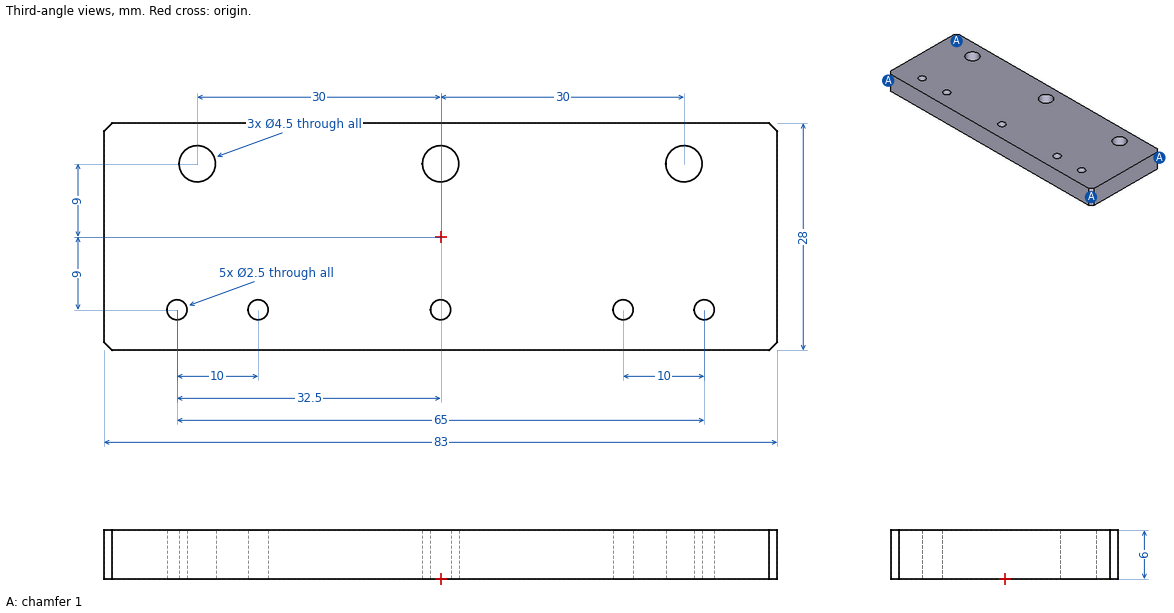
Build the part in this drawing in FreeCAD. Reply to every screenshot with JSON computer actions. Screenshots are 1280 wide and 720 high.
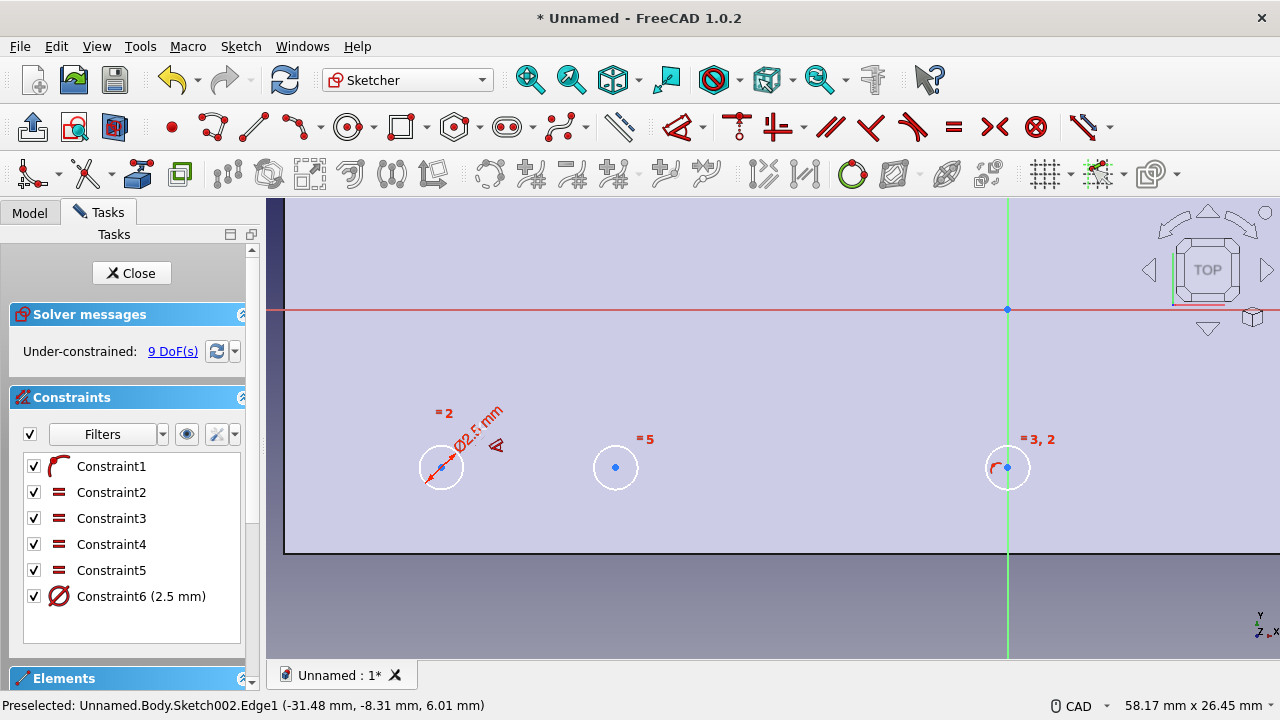
{"action": "left_click", "coordinate": [441, 468]}
{"action": "left_click", "coordinate": [407, 389]}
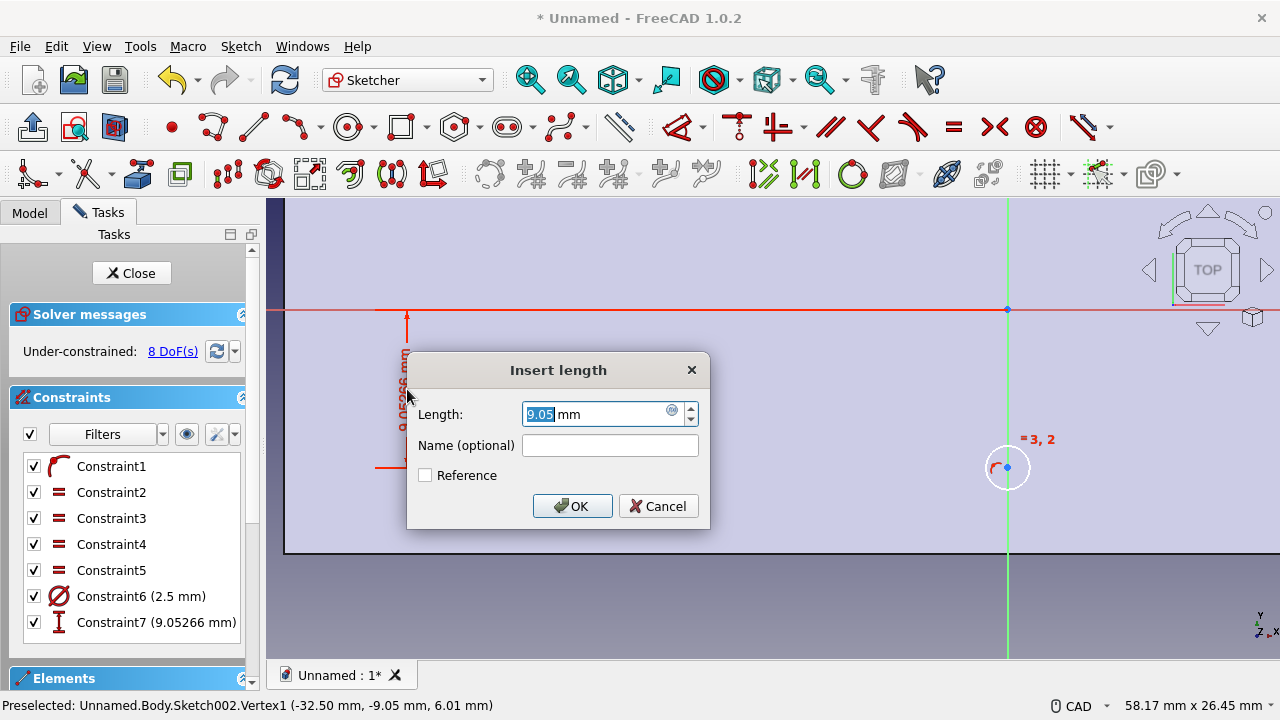
{"action": "type", "text": "9"}
{"action": "key", "text": "Return"}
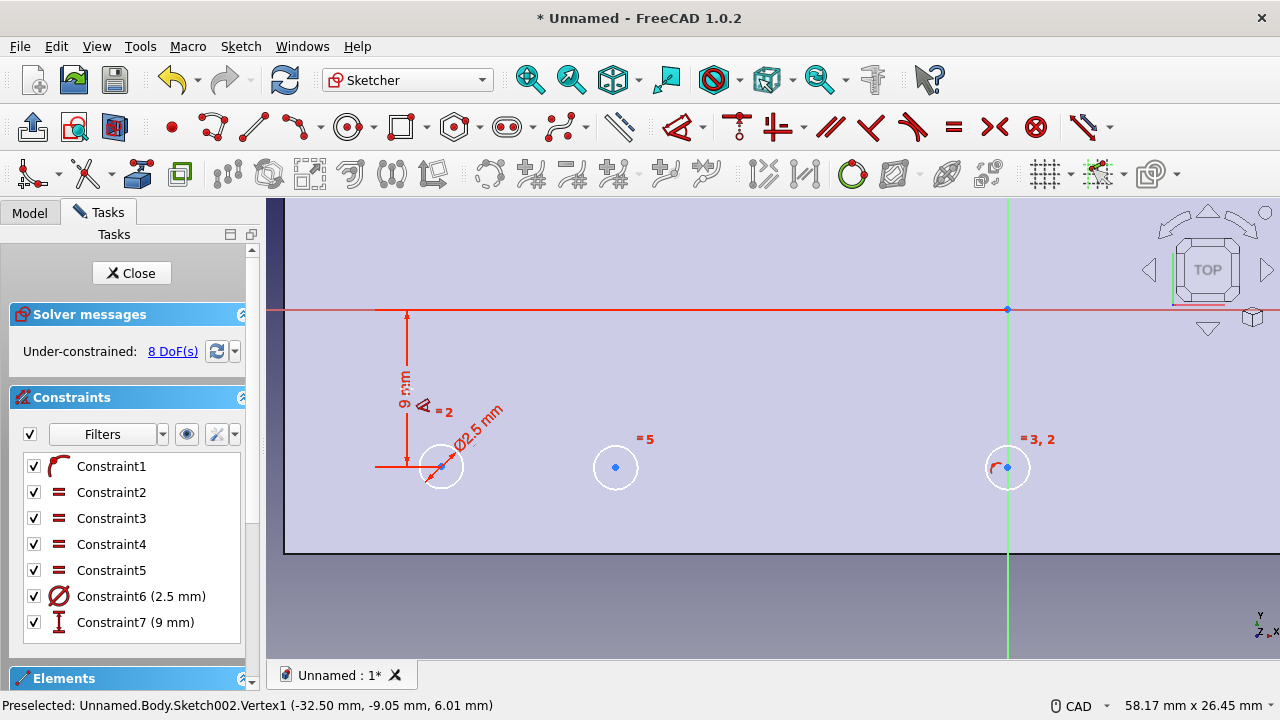
{"action": "left_click", "coordinate": [1008, 468]}
{"action": "left_click", "coordinate": [1042, 389]}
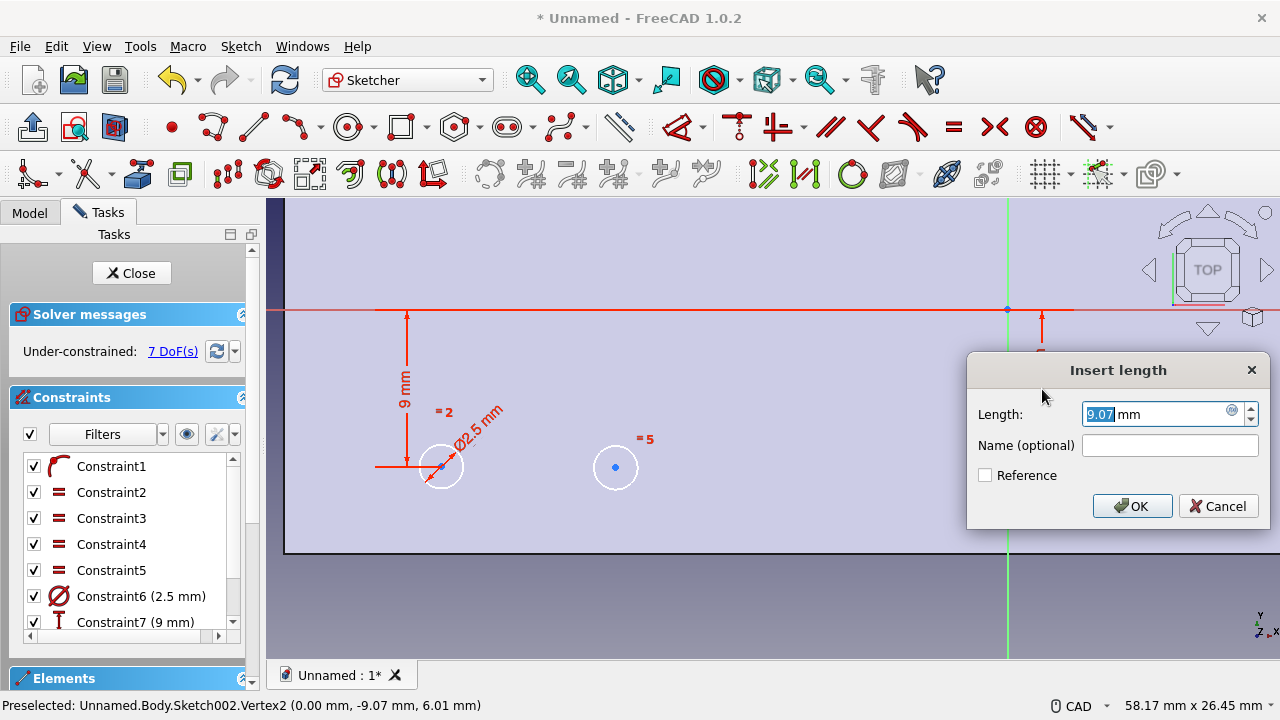
{"action": "type", "text": "9"}
{"action": "key", "text": "Return"}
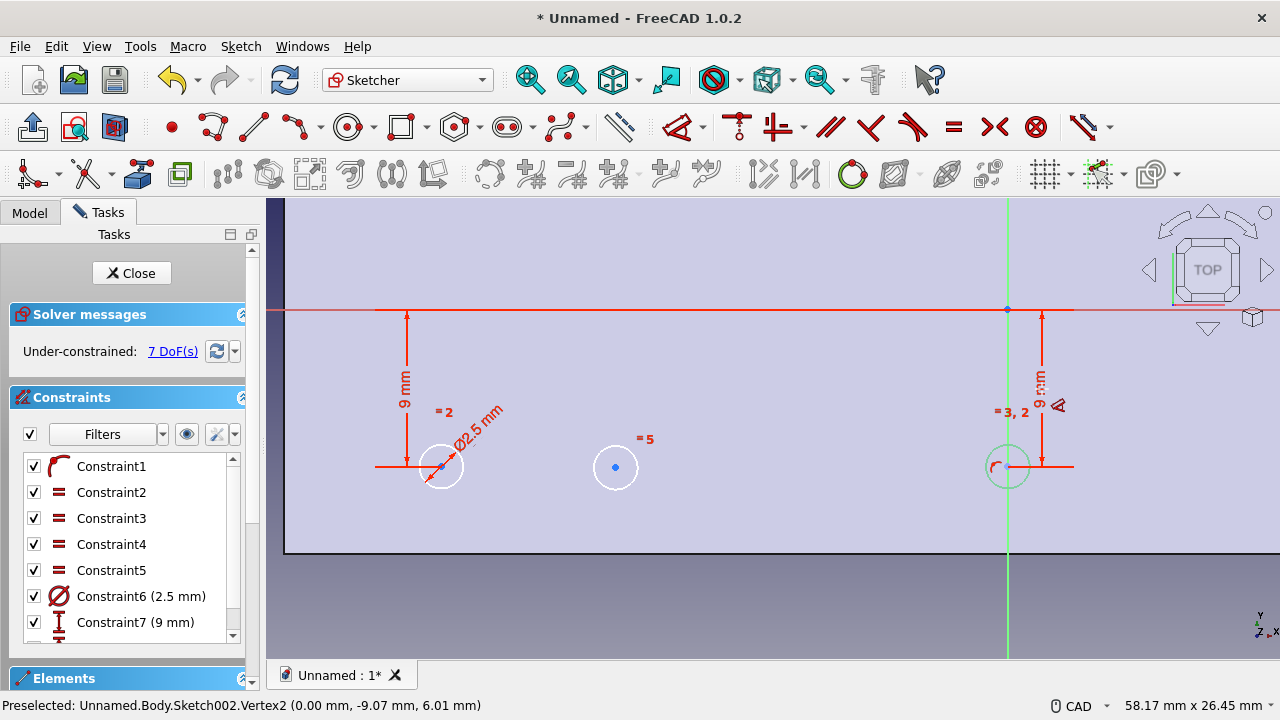
{"action": "scroll", "coordinate": [457, 452], "scroll_direction": "down", "scroll_amount": 4}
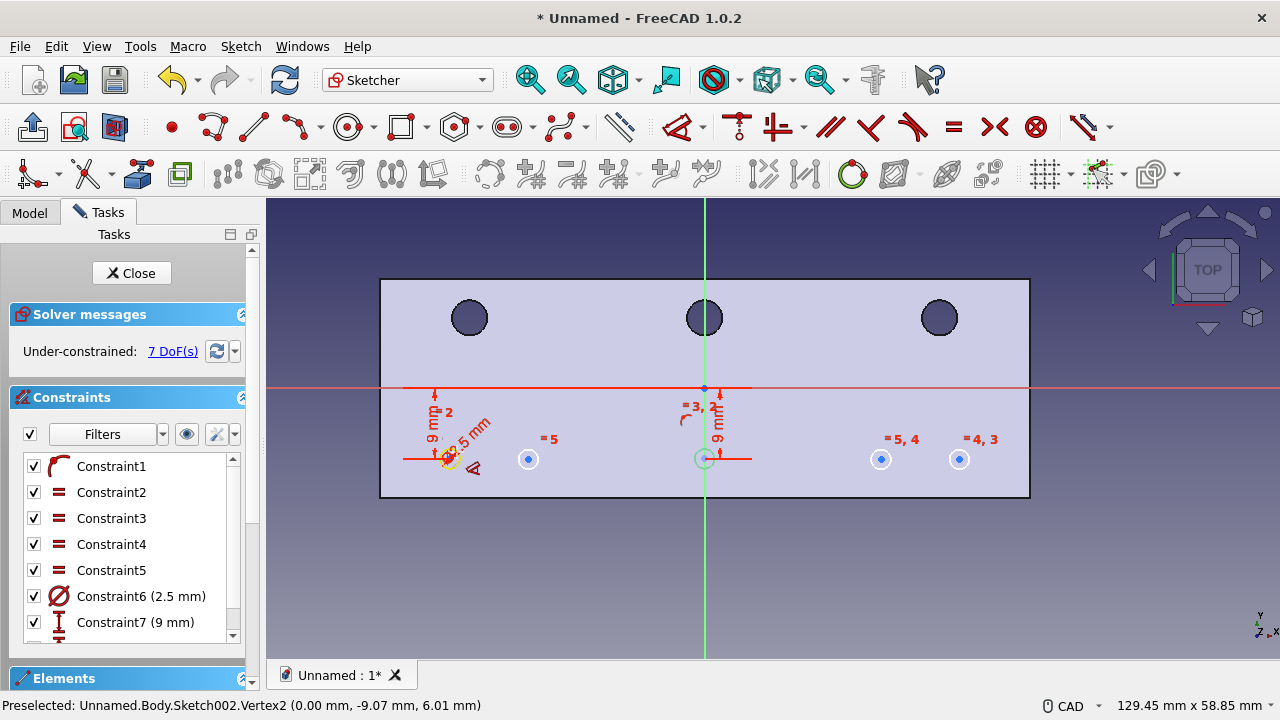
{"action": "left_click", "coordinate": [959, 459]}
{"action": "left_click", "coordinate": [993, 424]}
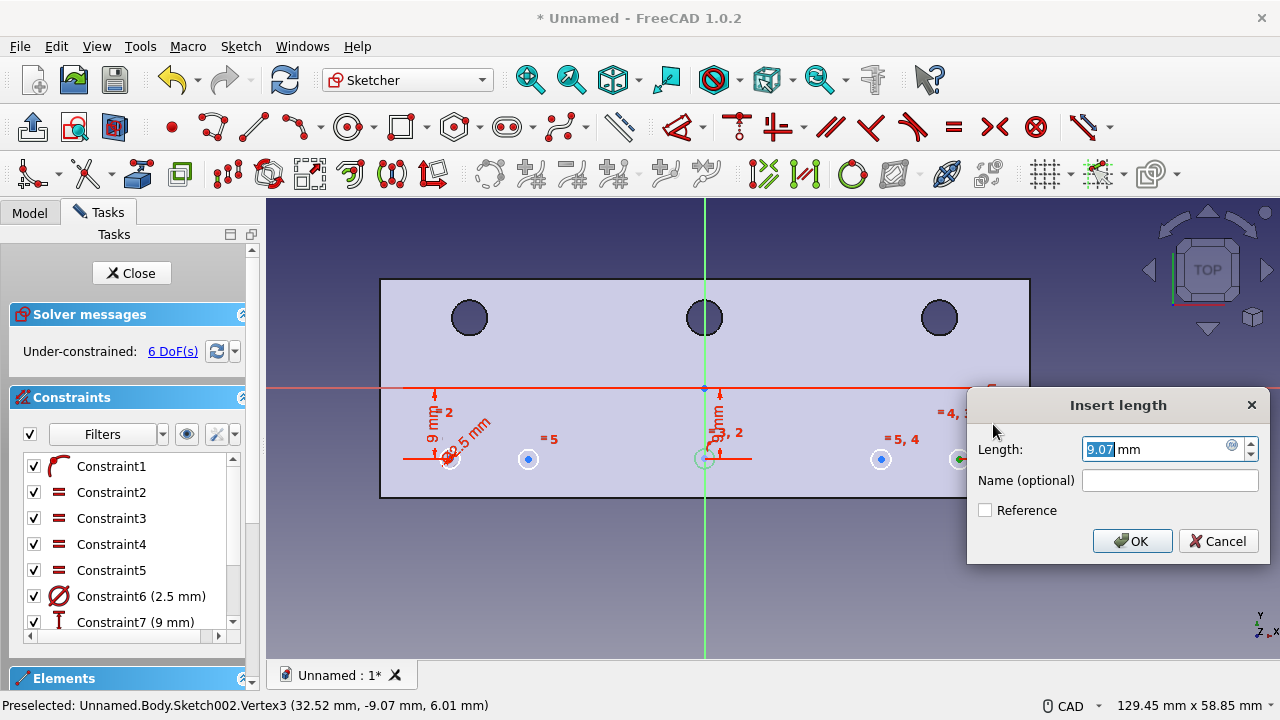
{"action": "type", "text": "9"}
{"action": "key", "text": "Return"}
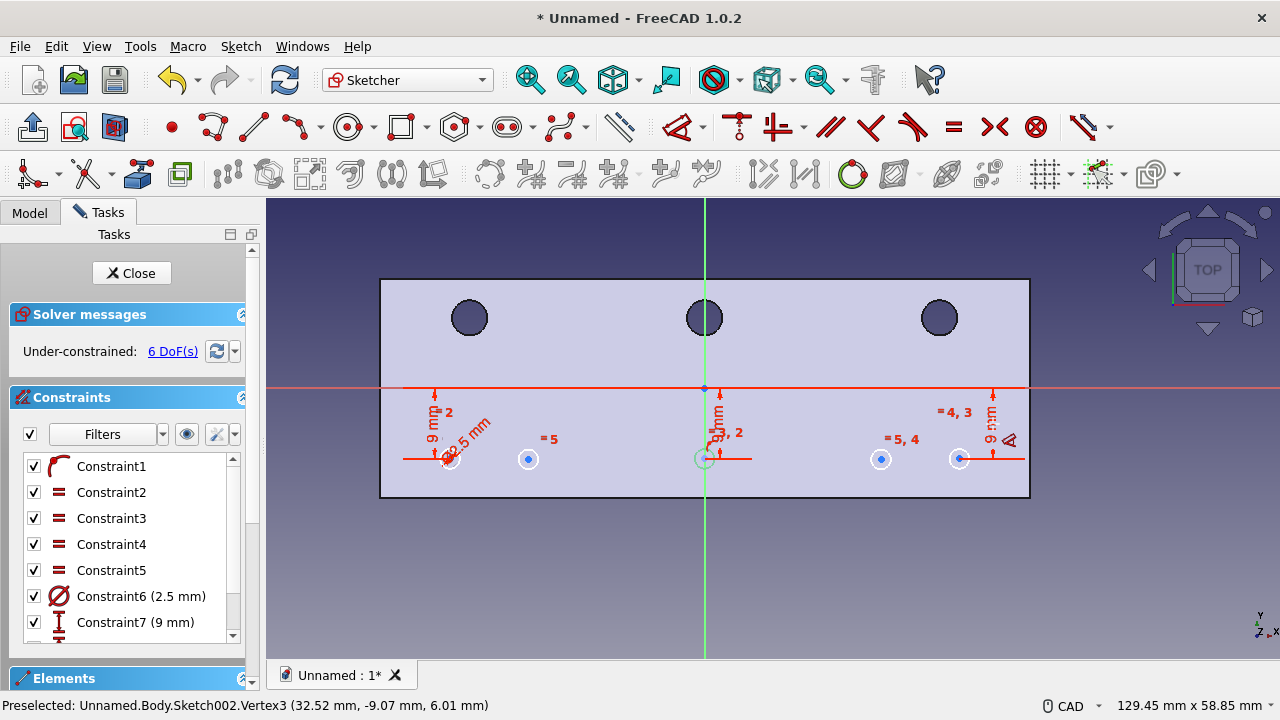
{"action": "left_click", "coordinate": [881, 459]}
{"action": "left_click", "coordinate": [915, 424]}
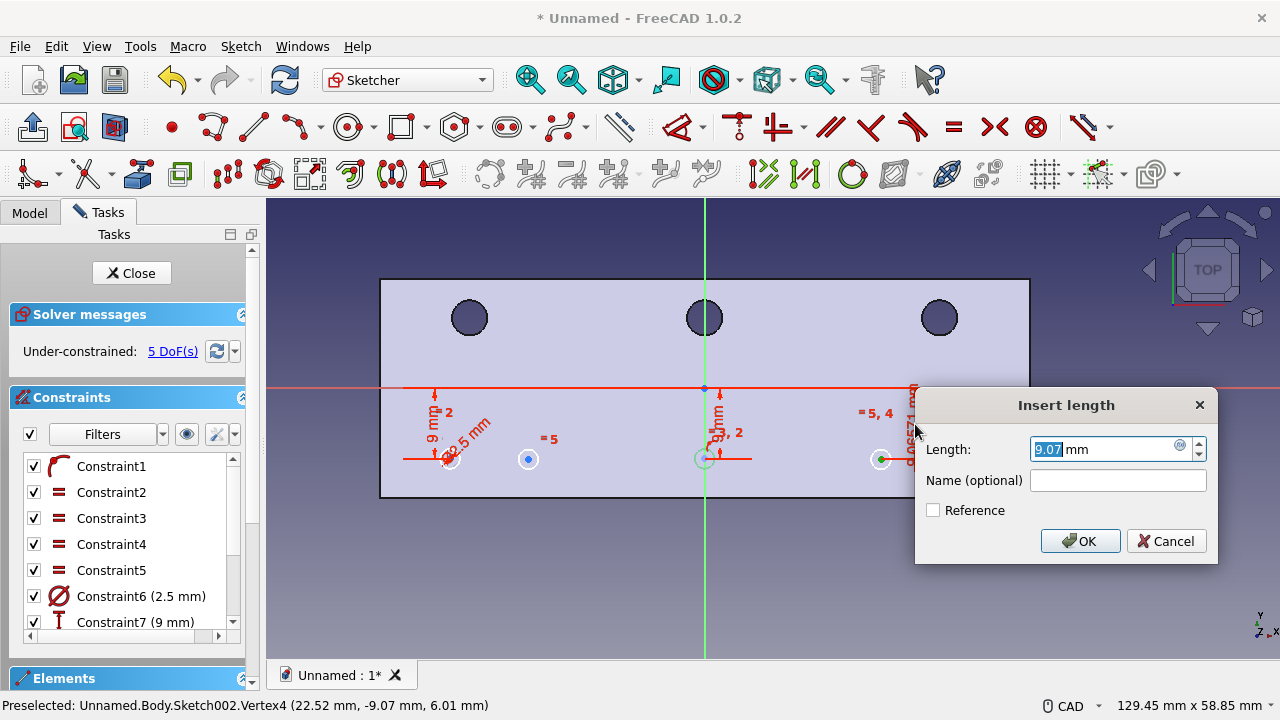
{"action": "type", "text": "9"}
{"action": "key", "text": "Return"}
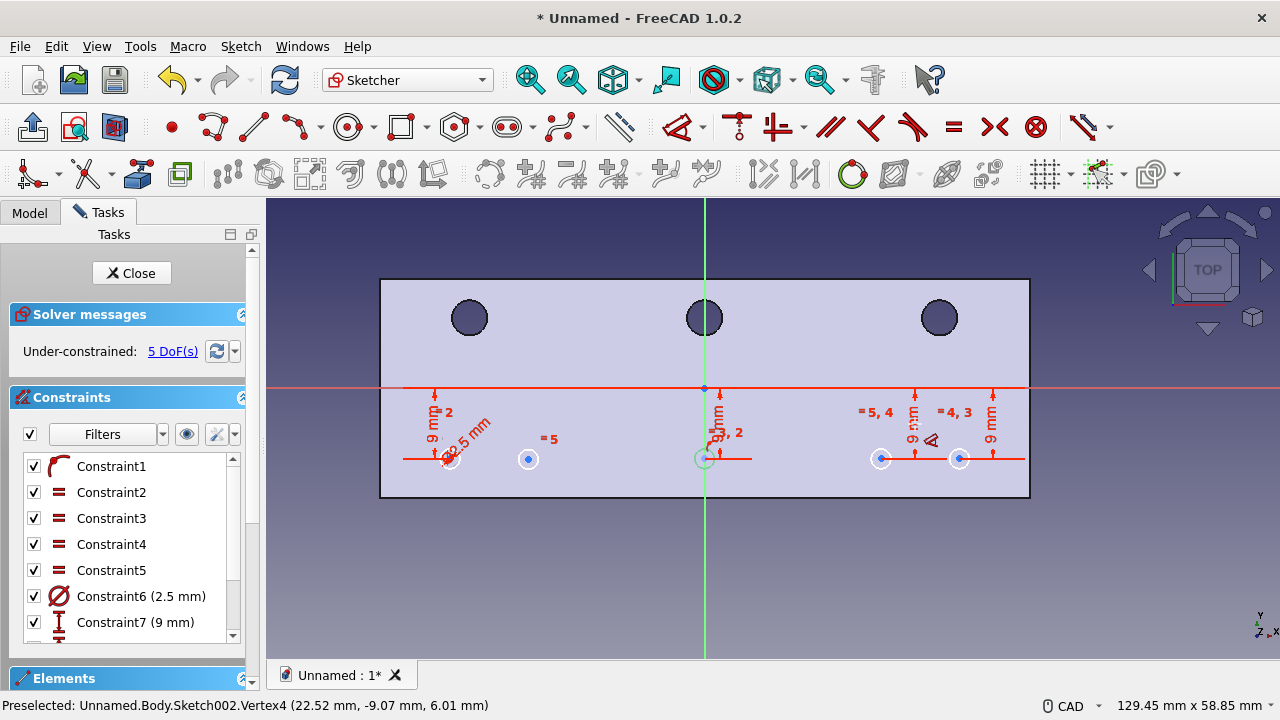
{"action": "left_click", "coordinate": [528, 459]}
{"action": "left_click", "coordinate": [739, 449]}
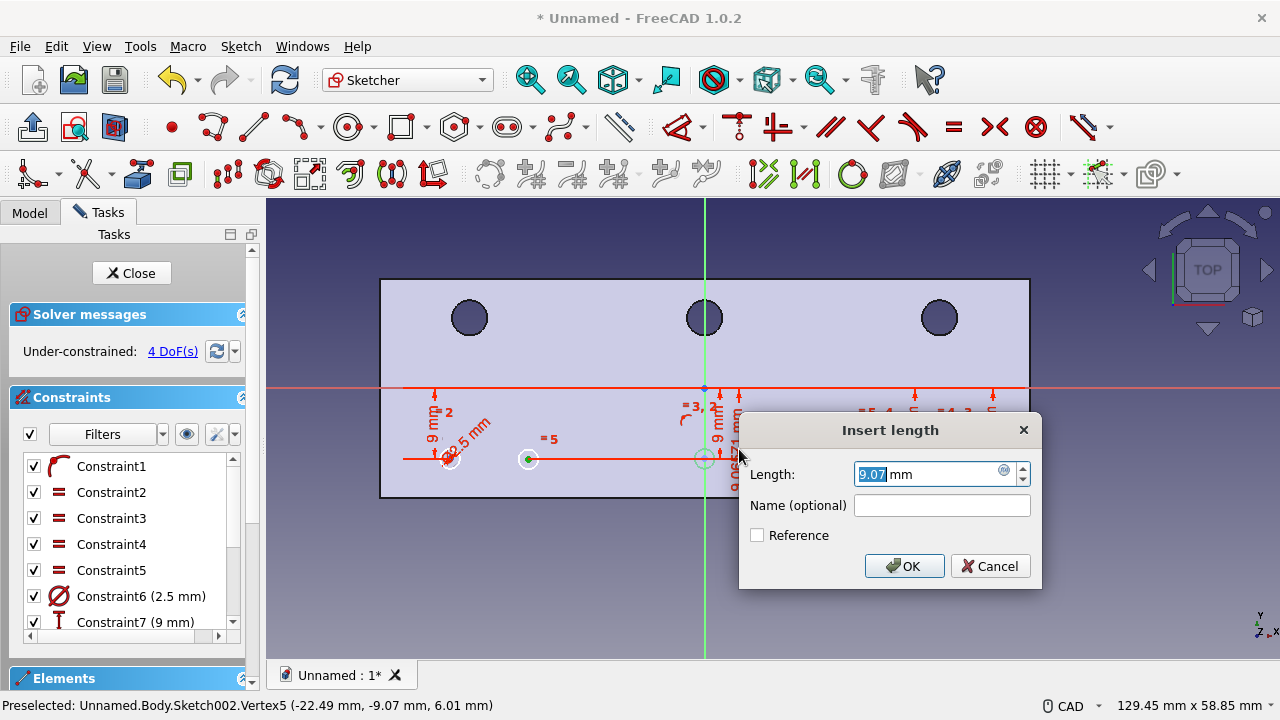
{"action": "type", "text": "9"}
{"action": "key", "text": "Return"}